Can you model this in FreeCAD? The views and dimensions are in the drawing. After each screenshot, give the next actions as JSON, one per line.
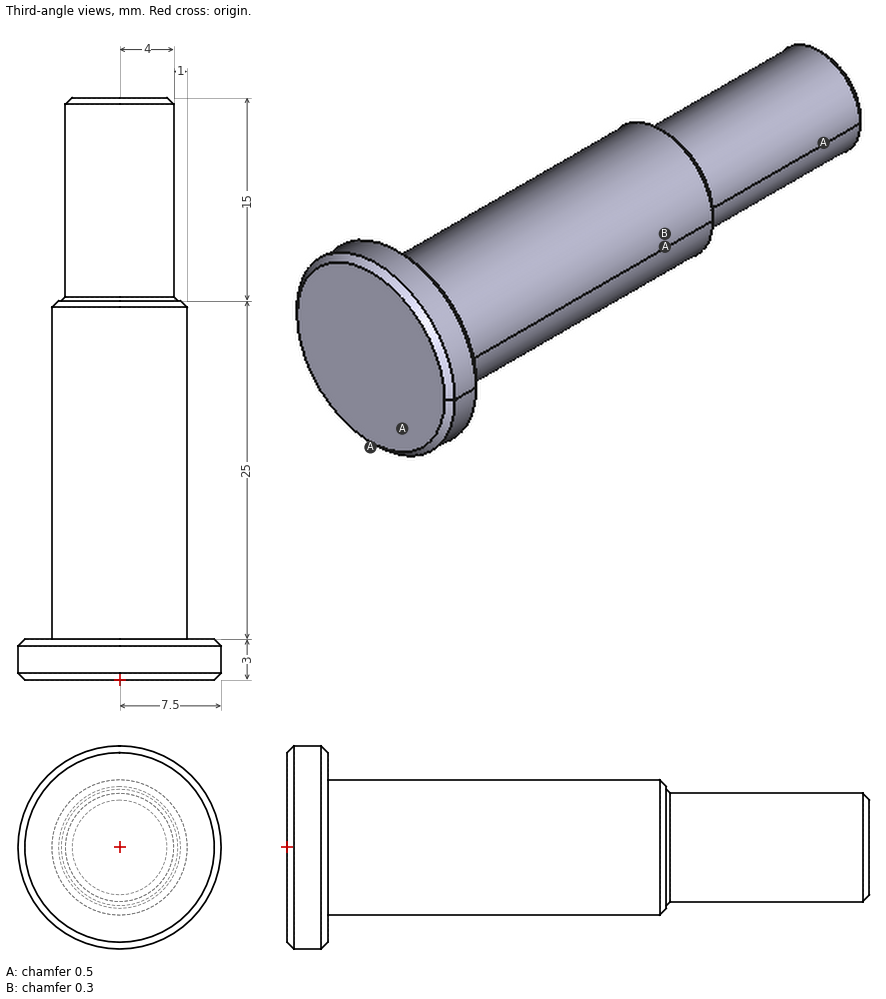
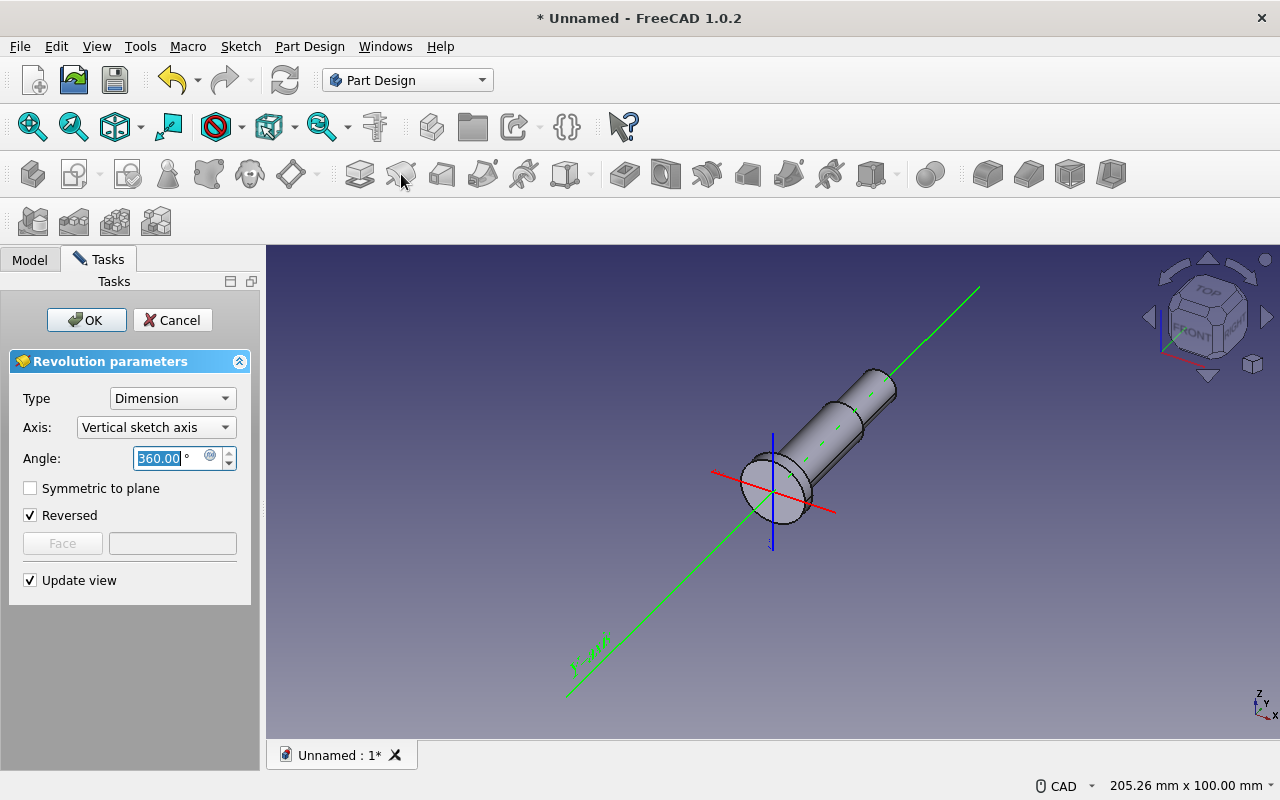
{"action": "left_click", "coordinate": [87, 320]}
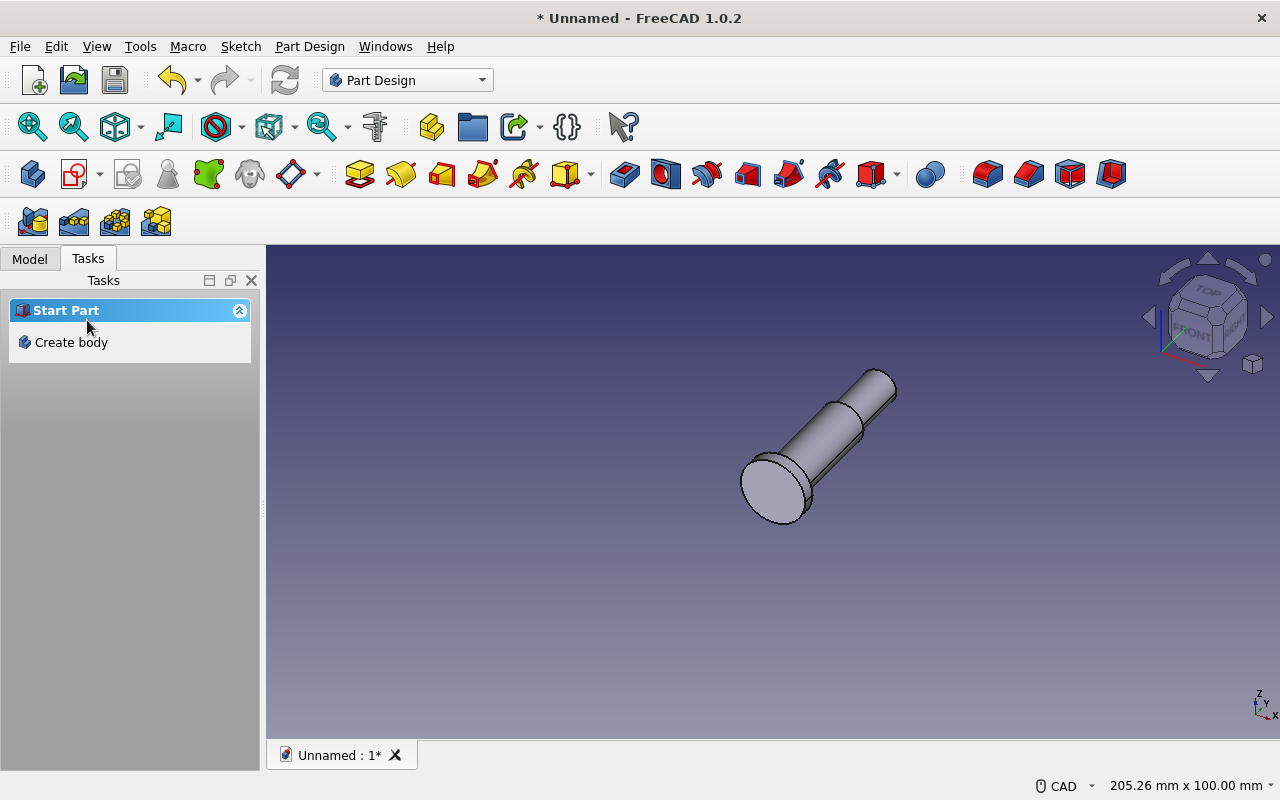
{"action": "left_click", "coordinate": [33, 128]}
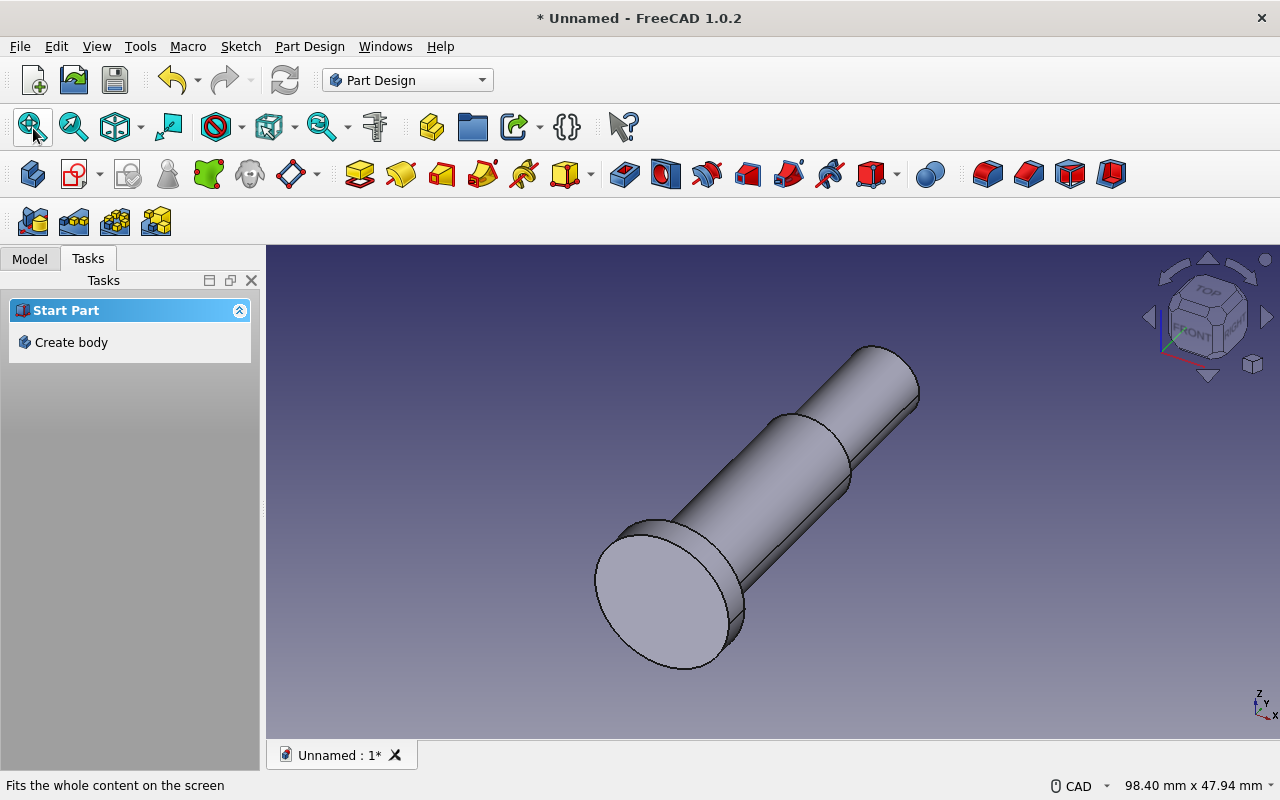
{"action": "left_click", "coordinate": [608, 546]}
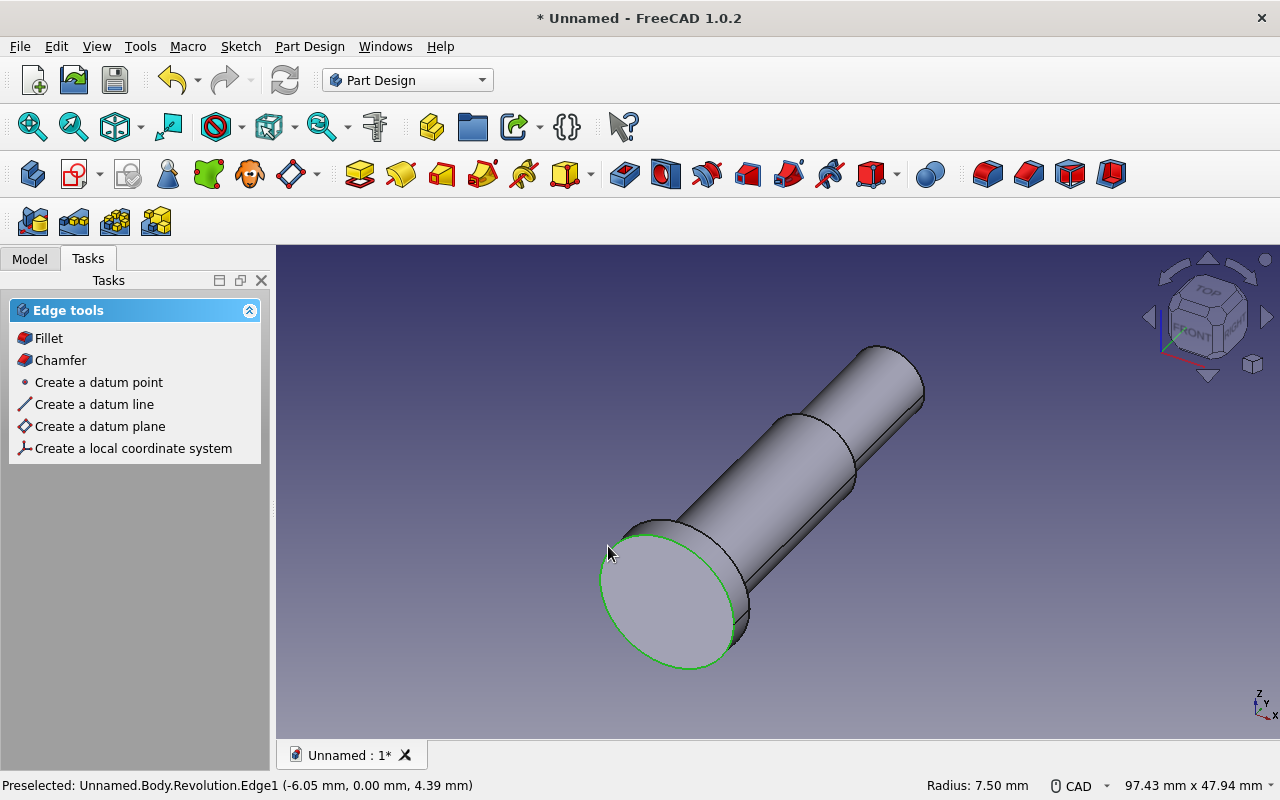
{"action": "key", "text": "0"}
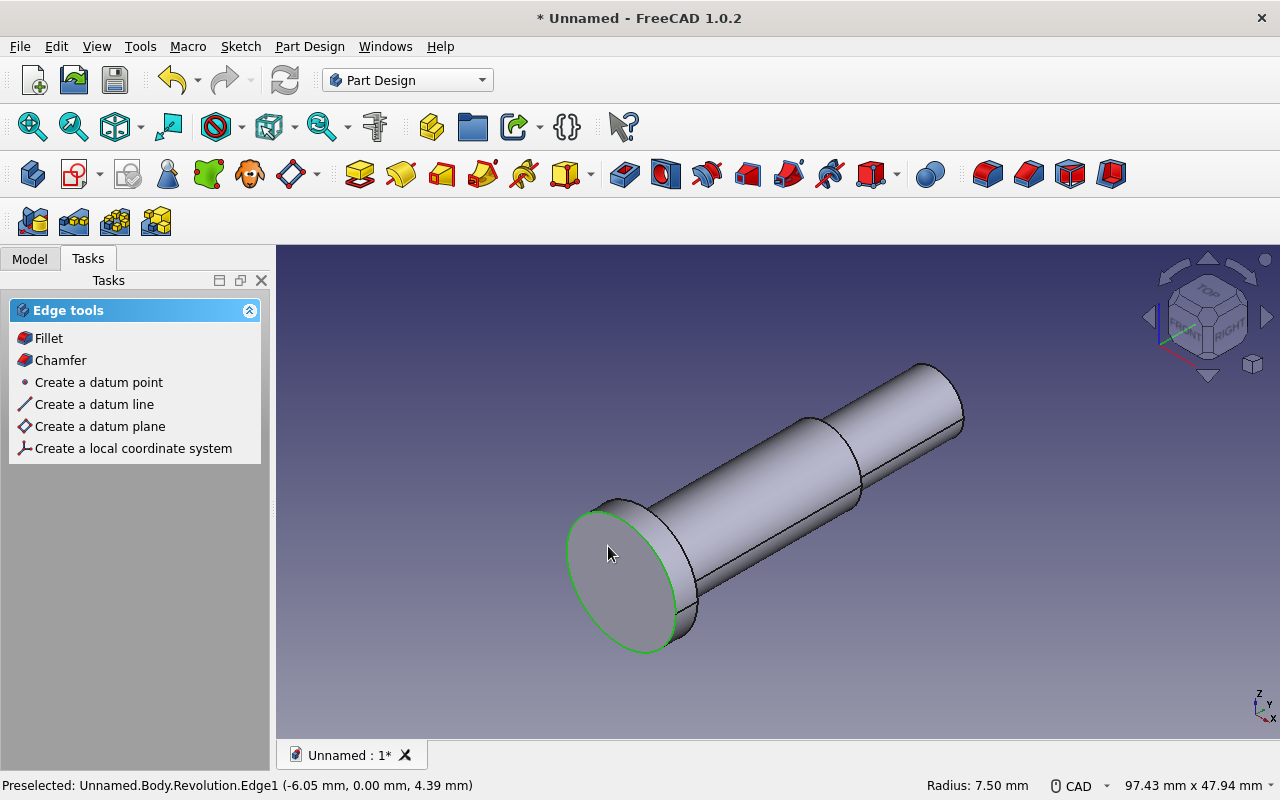
{"action": "left_click", "coordinate": [837, 430], "text": "ctrl"}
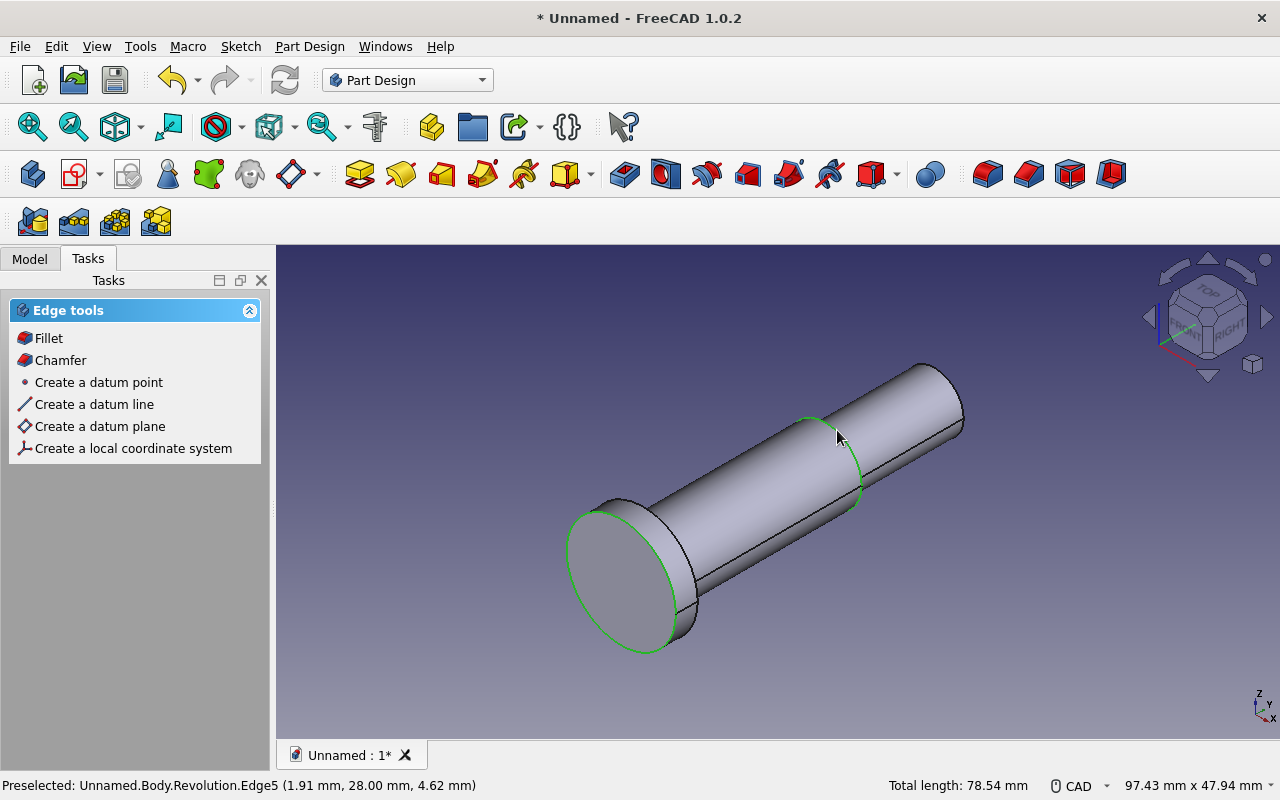
{"action": "key", "text": "2"}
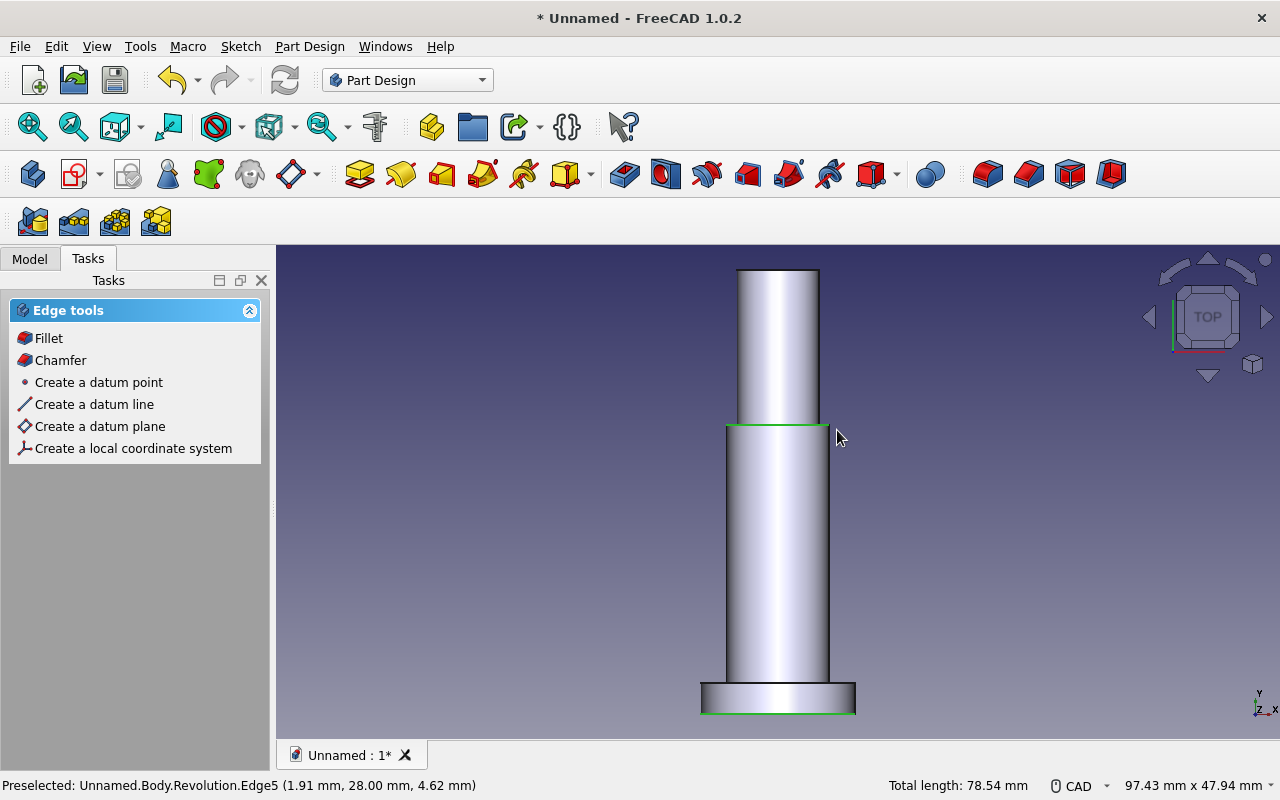
{"action": "left_click", "coordinate": [715, 682], "text": "ctrl"}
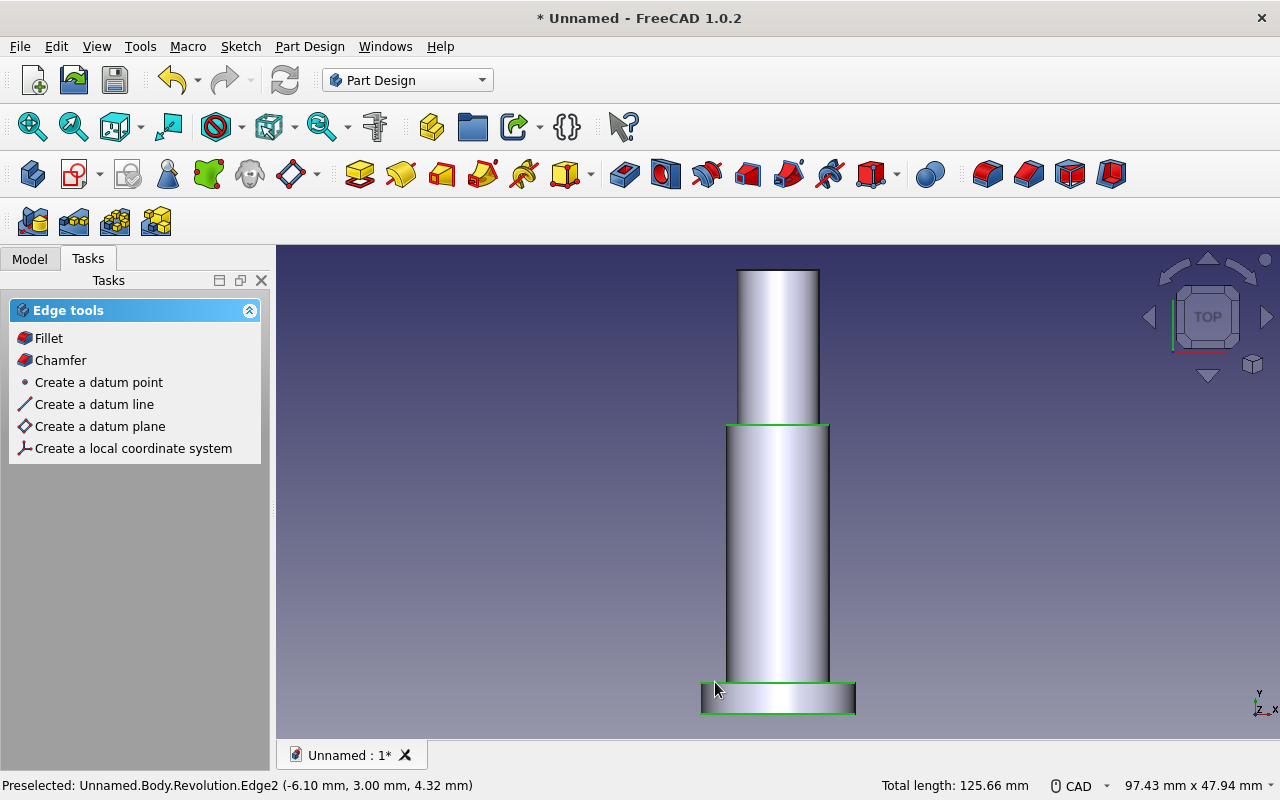
{"action": "key", "text": "1"}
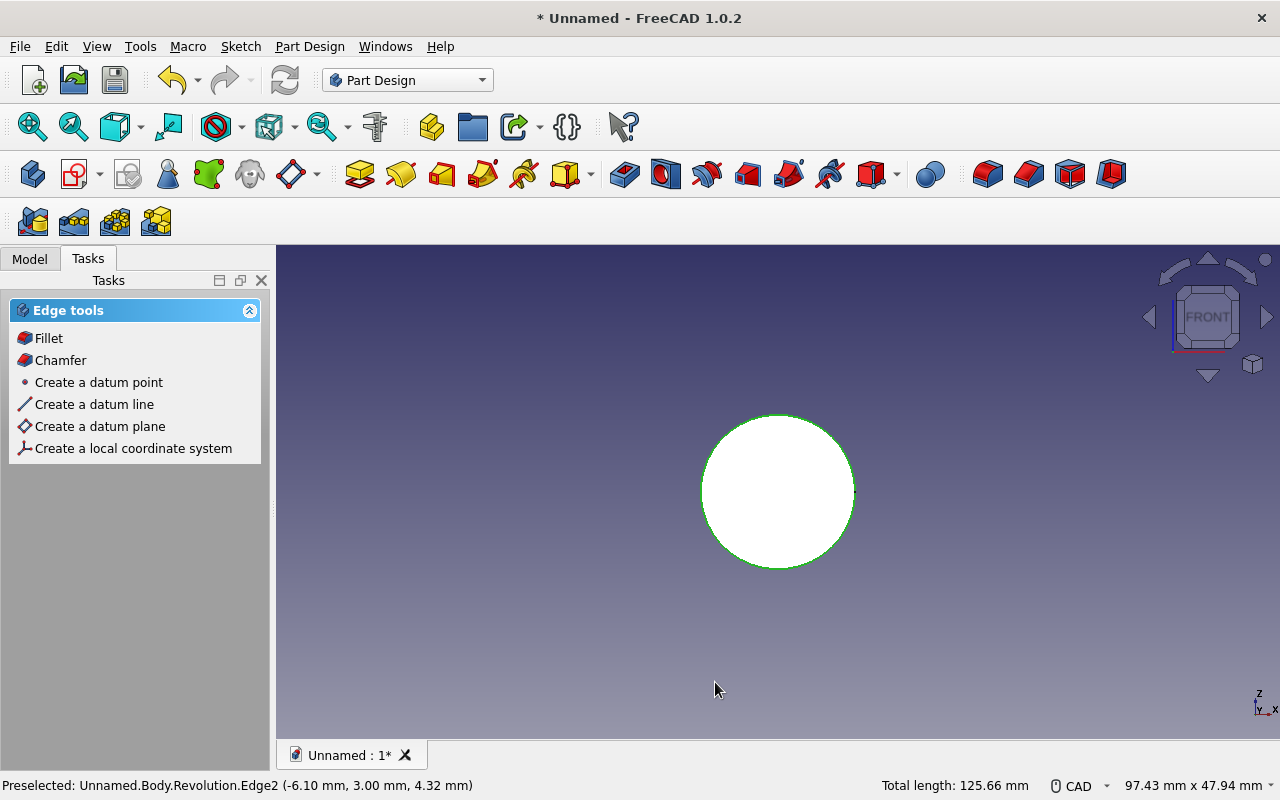
{"action": "left_click", "coordinate": [33, 128]}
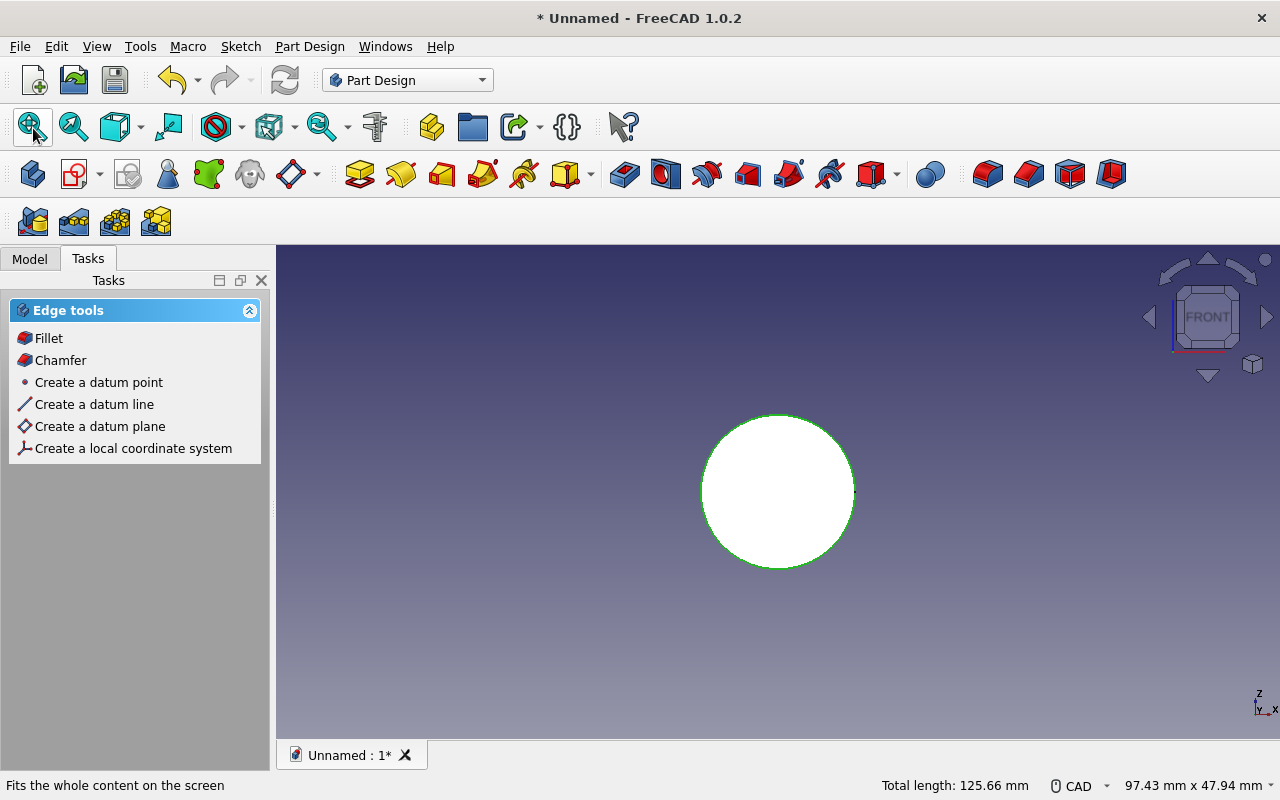
{"action": "key", "text": "3"}